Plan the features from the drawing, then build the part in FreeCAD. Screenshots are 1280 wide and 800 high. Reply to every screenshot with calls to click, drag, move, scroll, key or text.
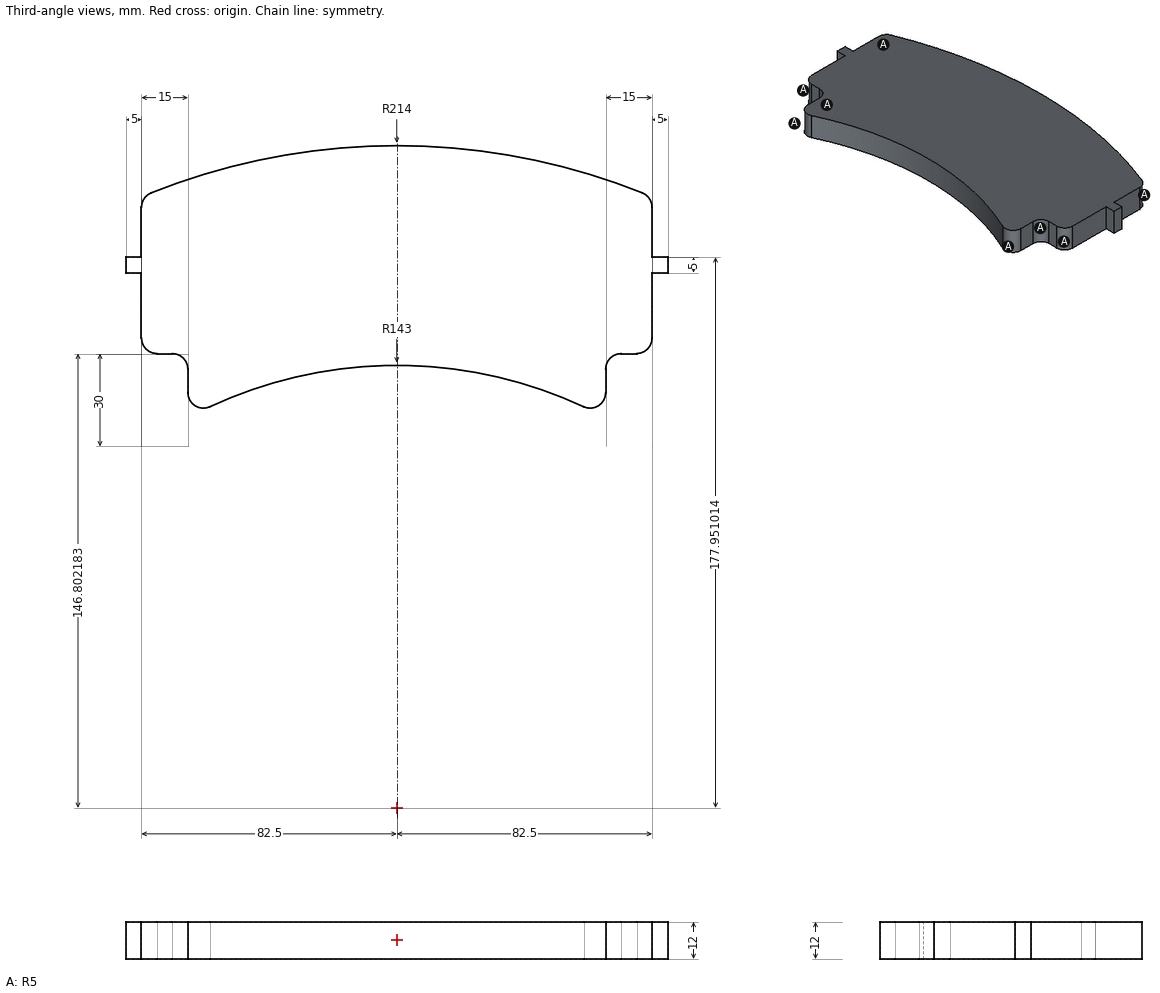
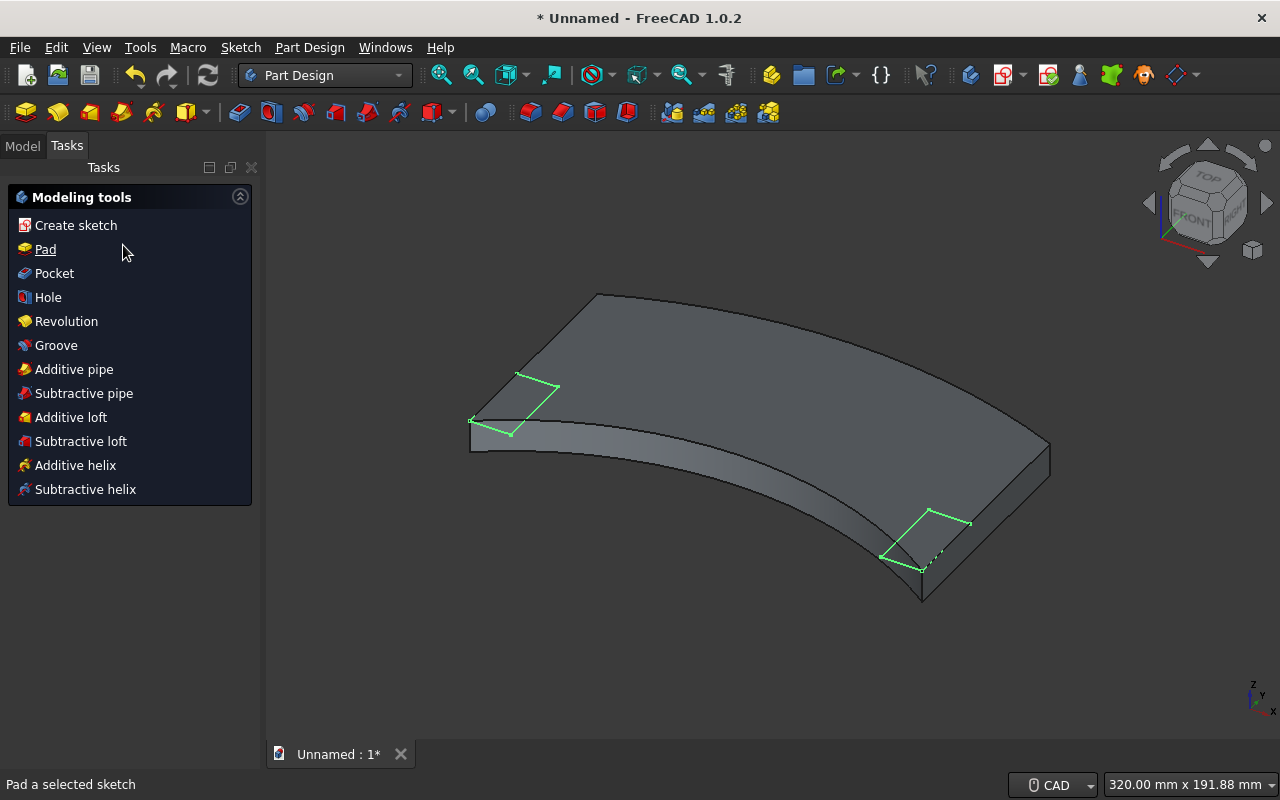
click(240, 112)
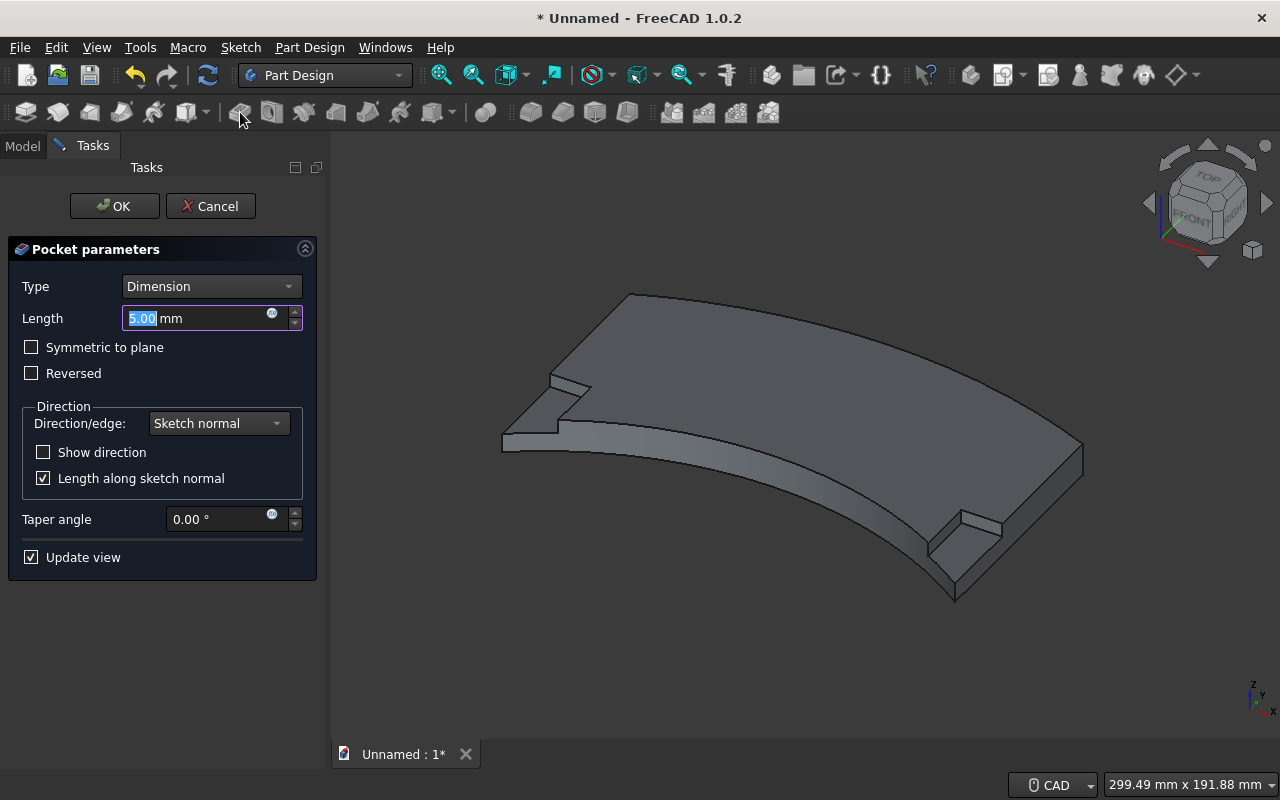
text(30)
key(Tab)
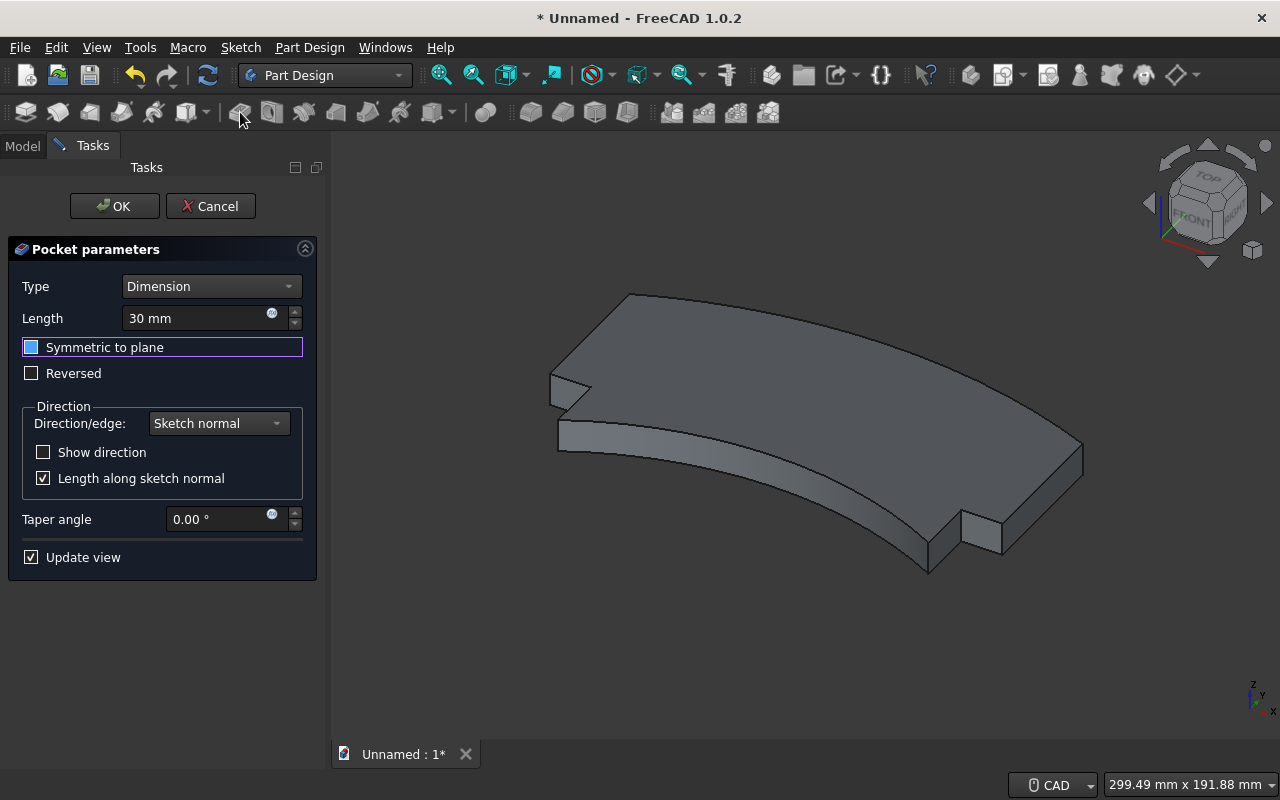
click(115, 206)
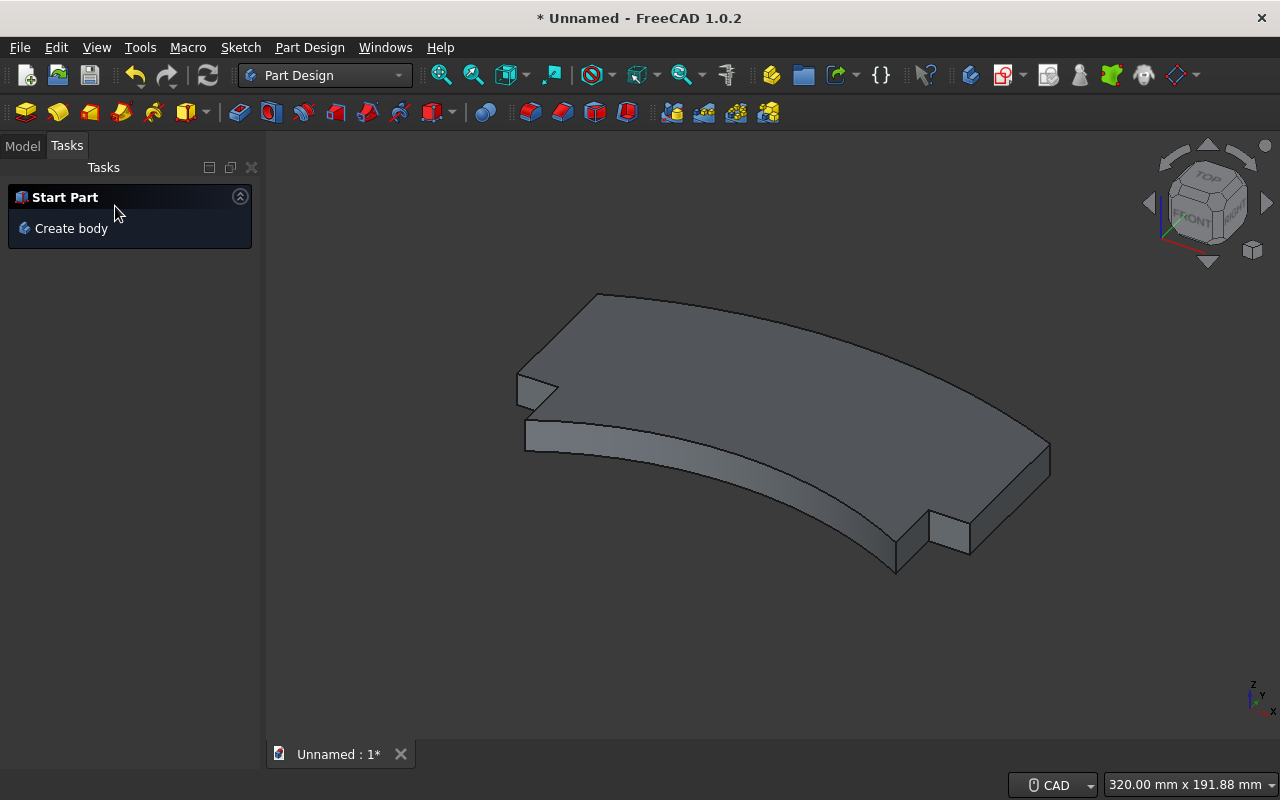
click(970, 538)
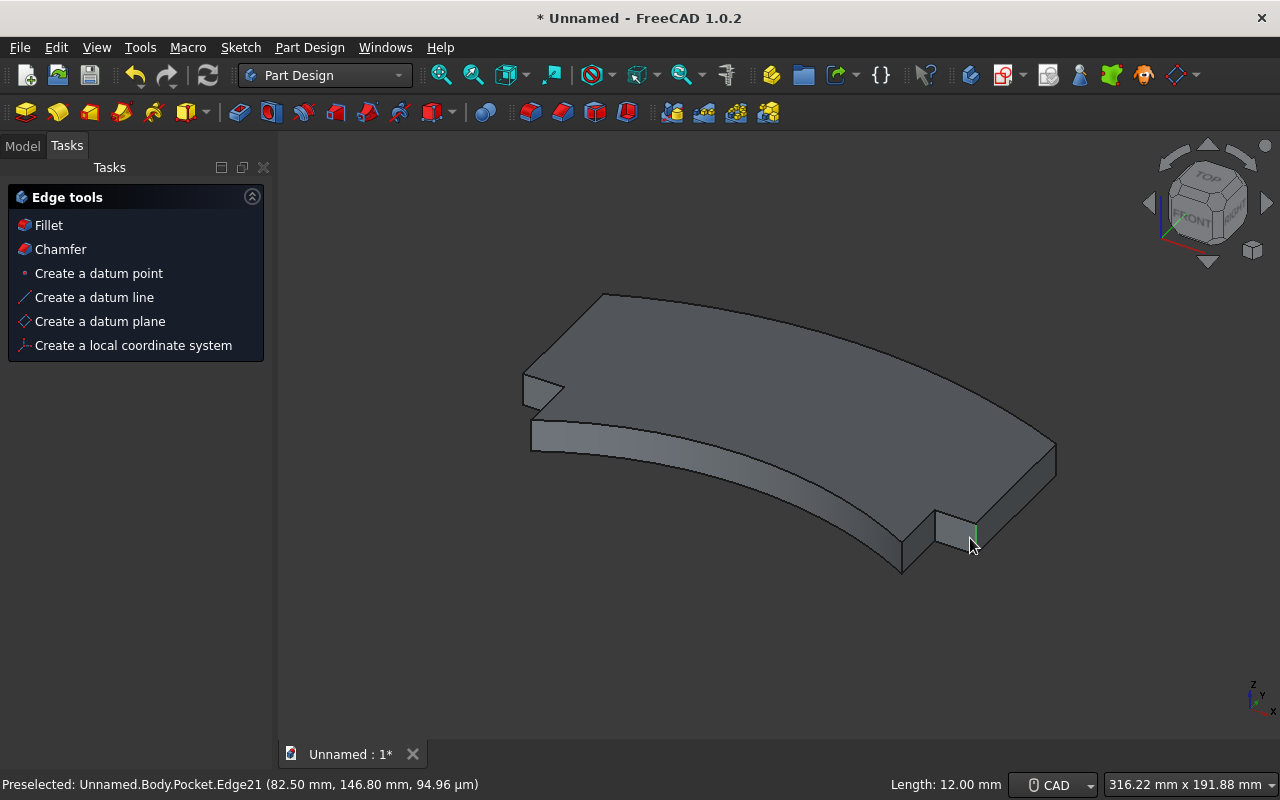
click(902, 557, ctrl)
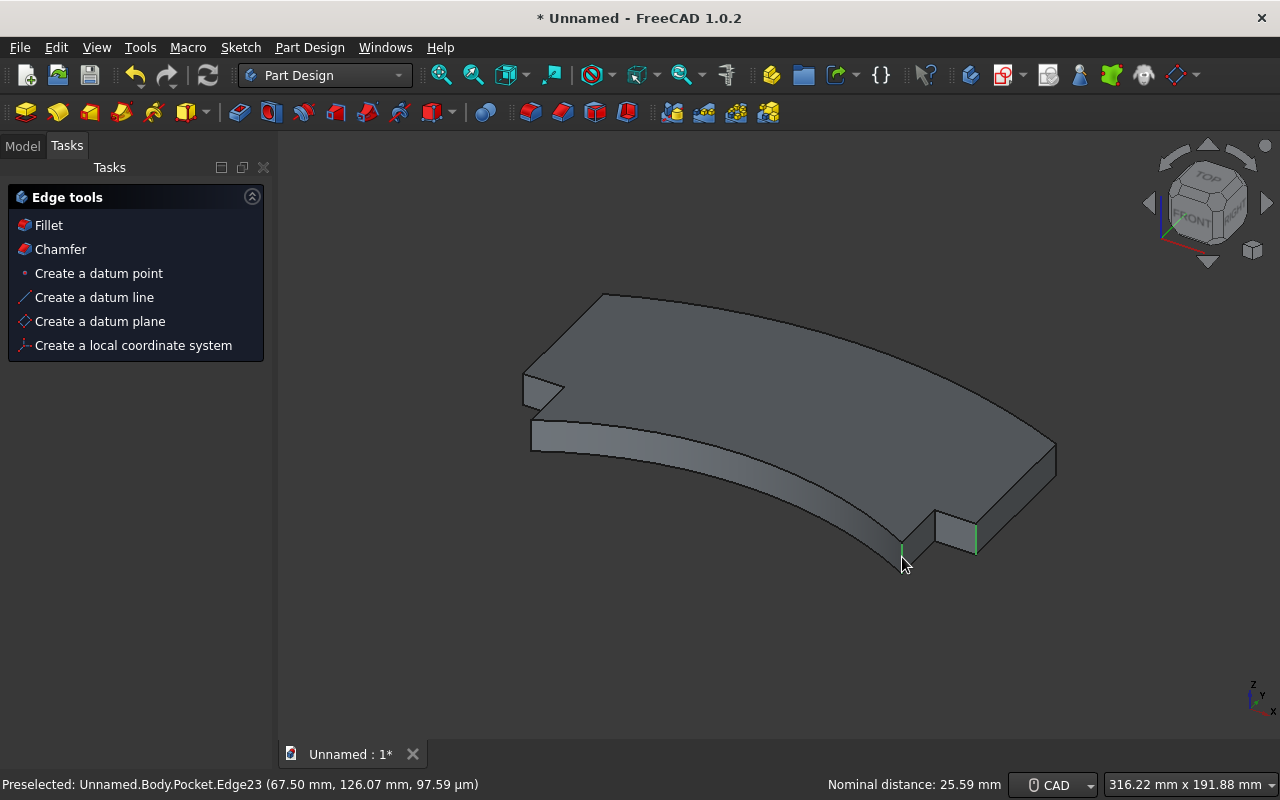
key(0)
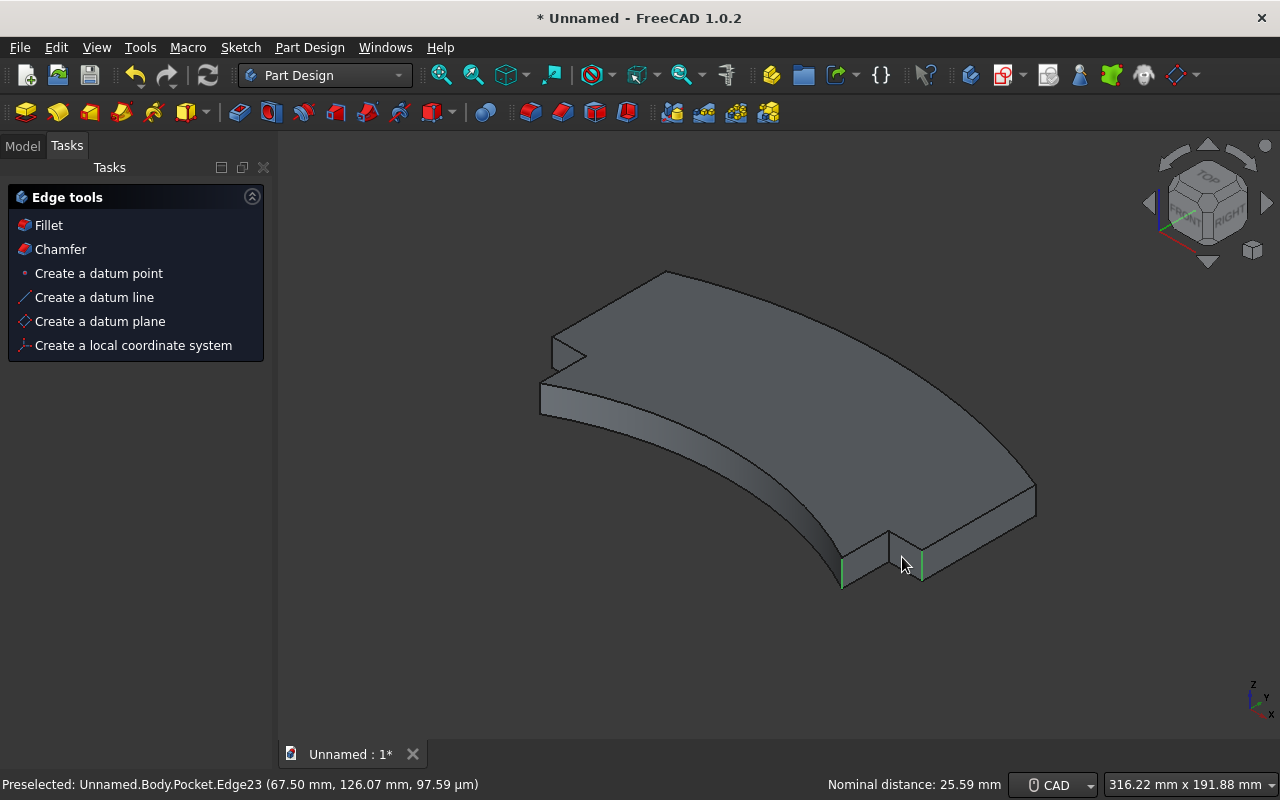
key(2)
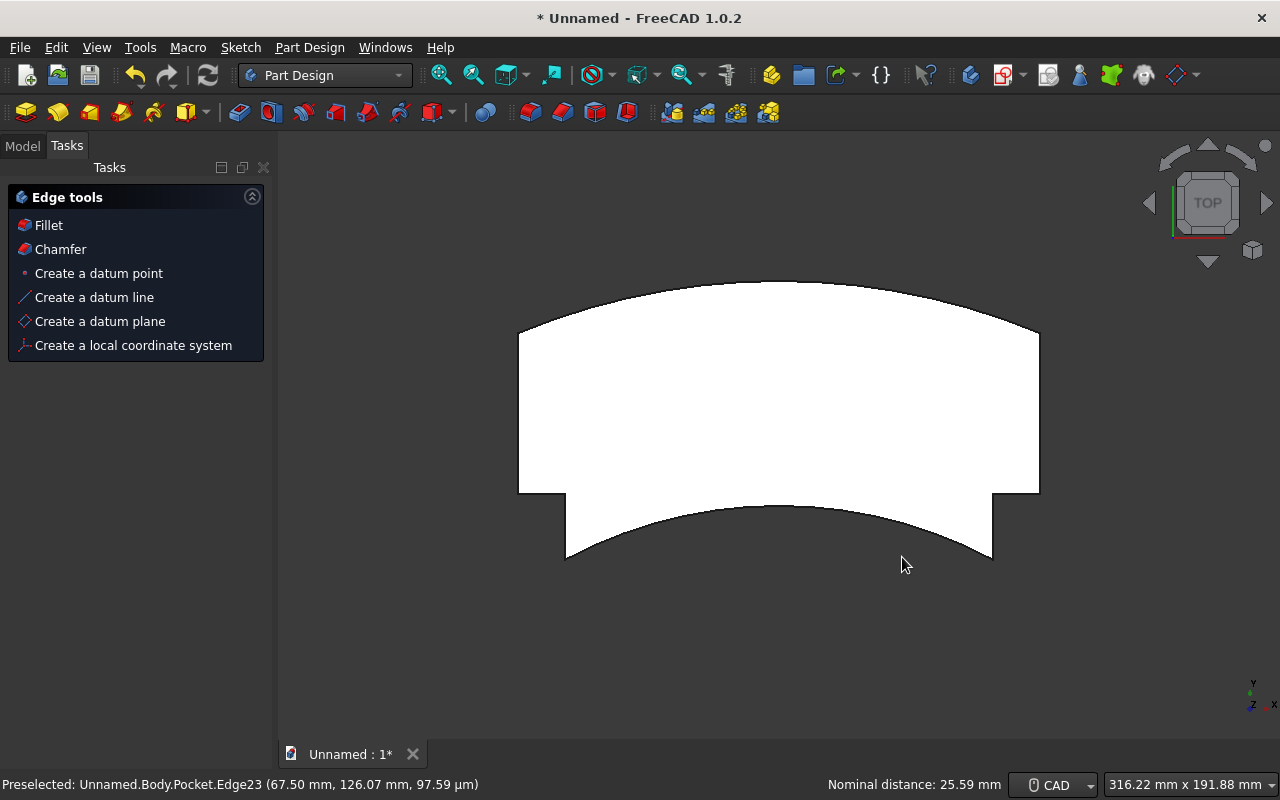
key(1)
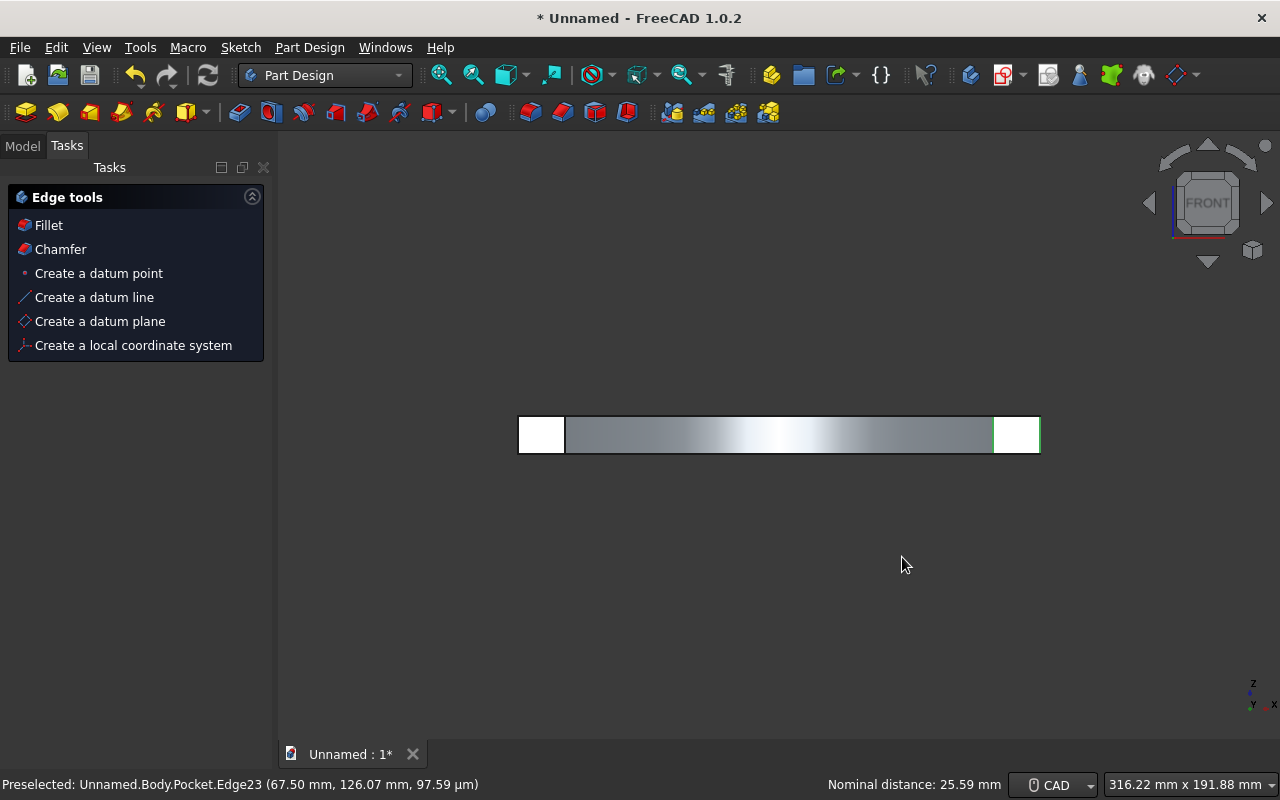
click(518, 434, ctrl)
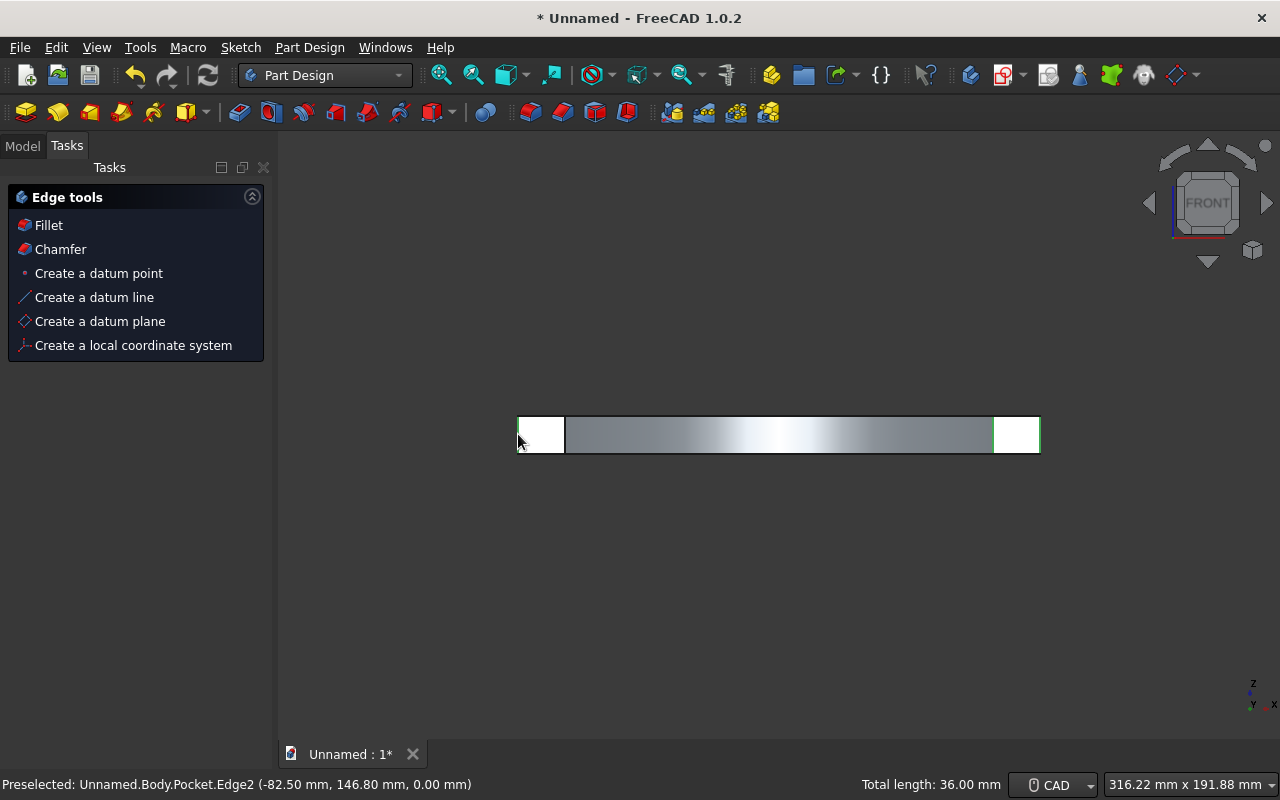
click(565, 434, ctrl)